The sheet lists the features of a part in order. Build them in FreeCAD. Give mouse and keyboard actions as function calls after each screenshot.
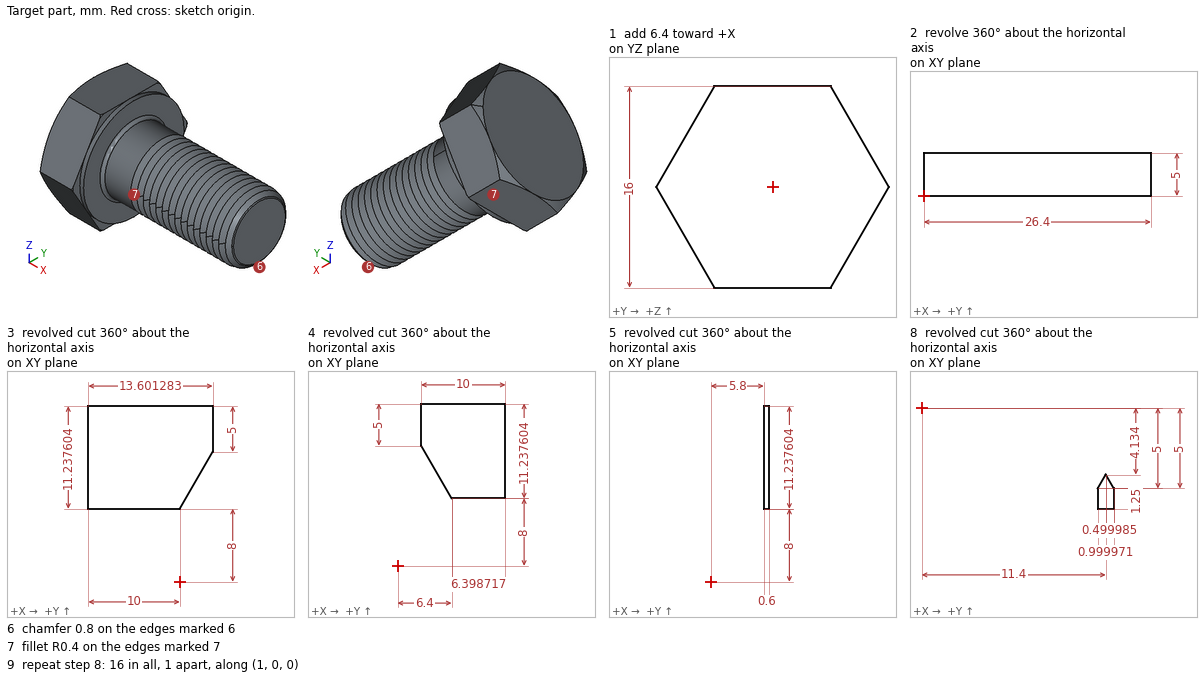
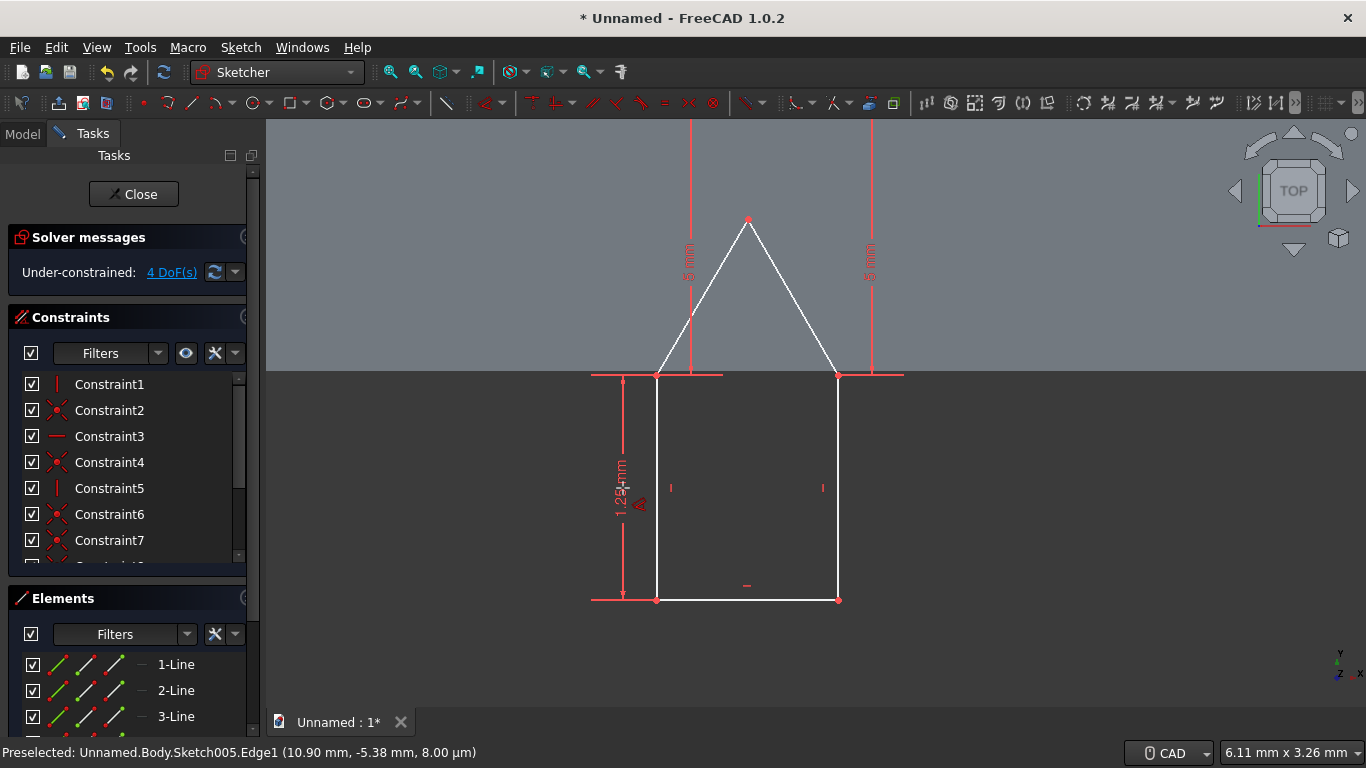
click(748, 220)
click(521, 254)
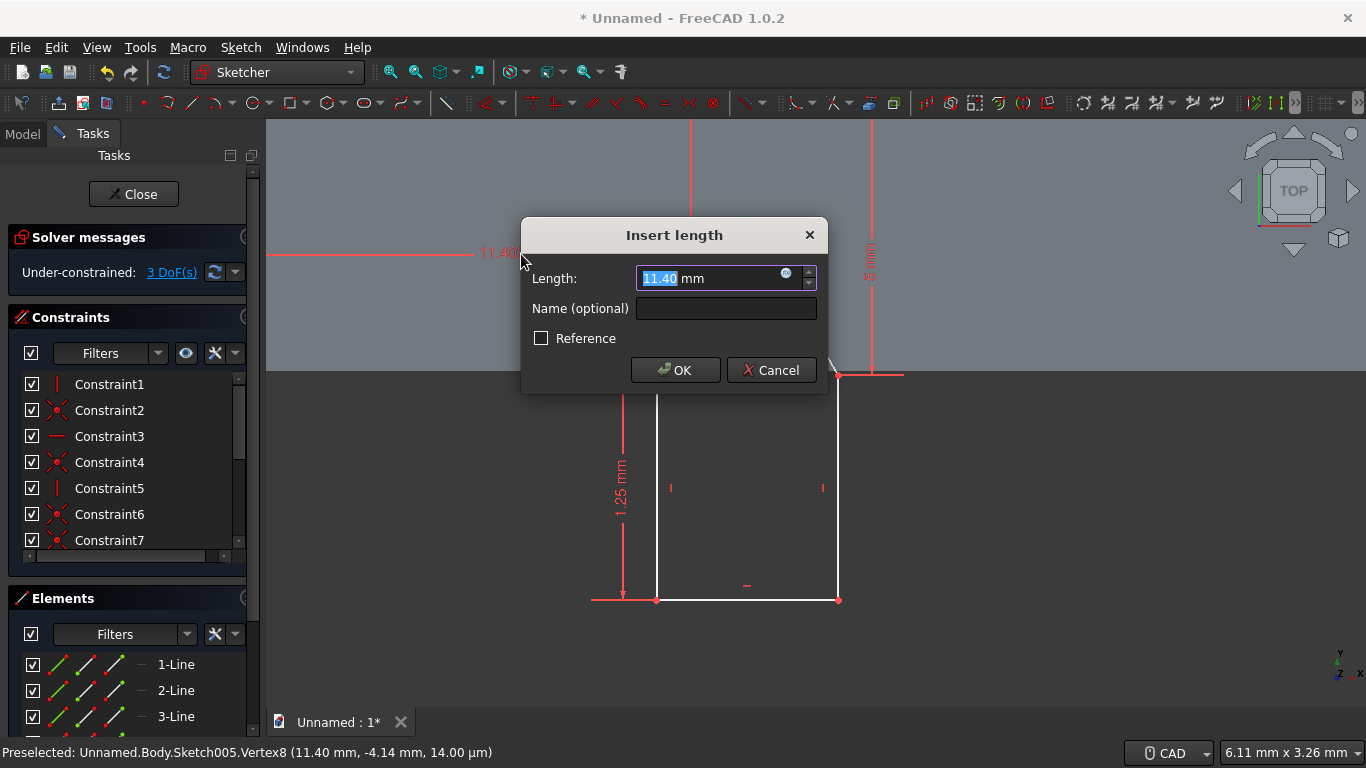
text(11.4)
key(Return)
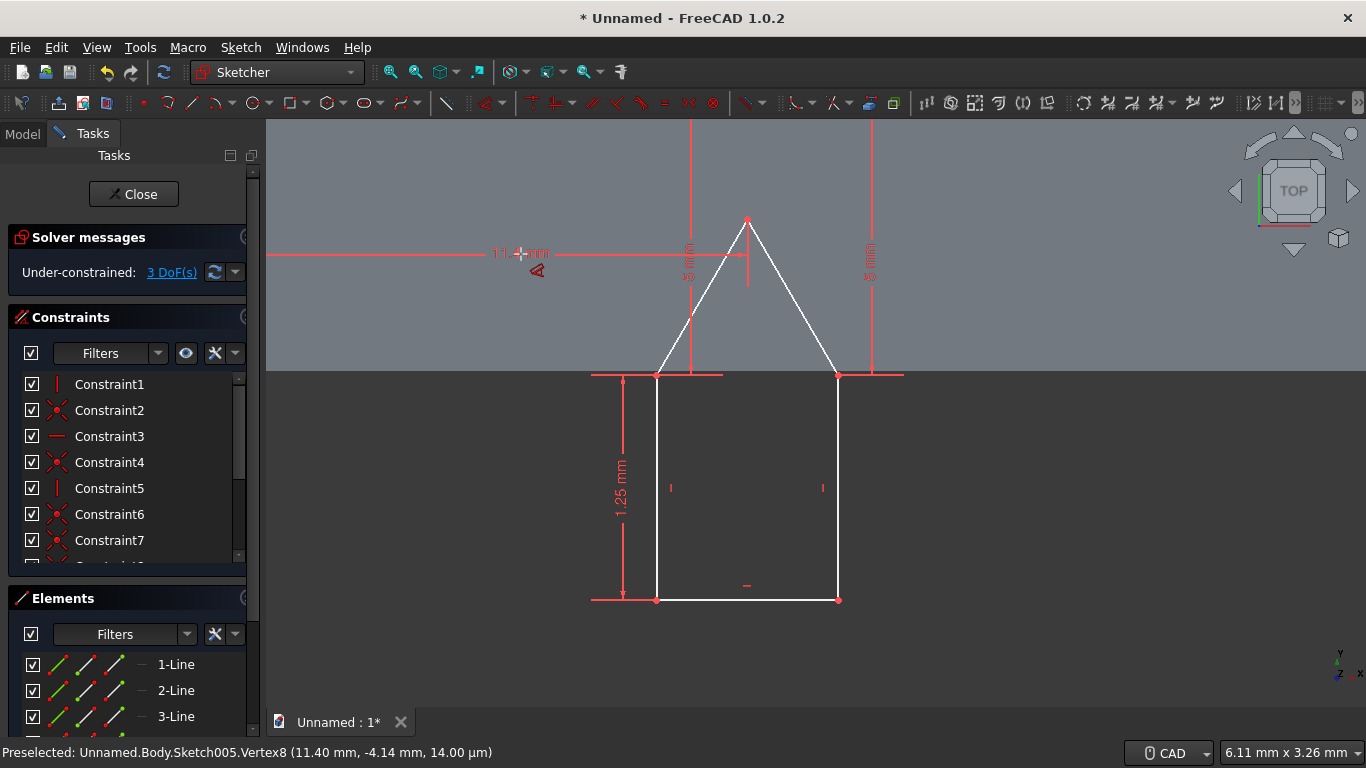
click(748, 220)
click(782, 183)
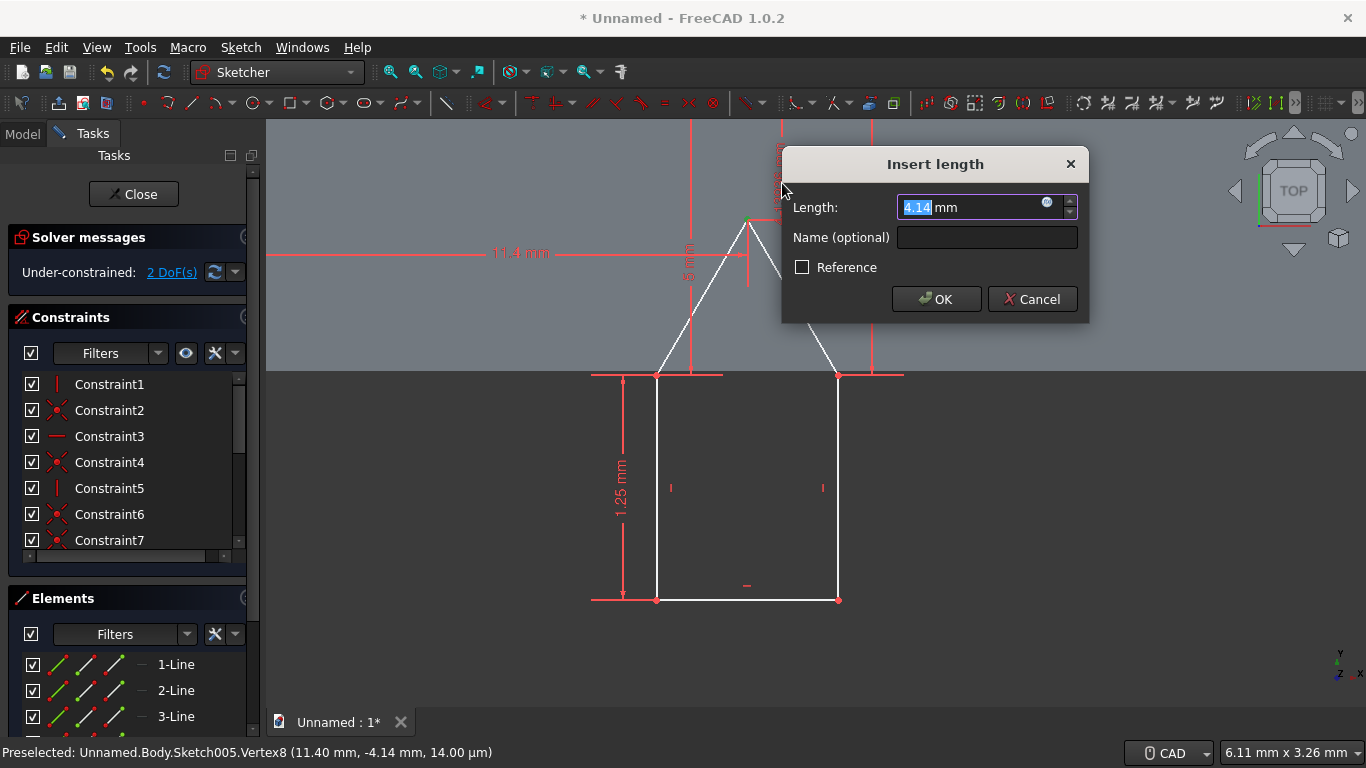
text(4.134)
key(Return)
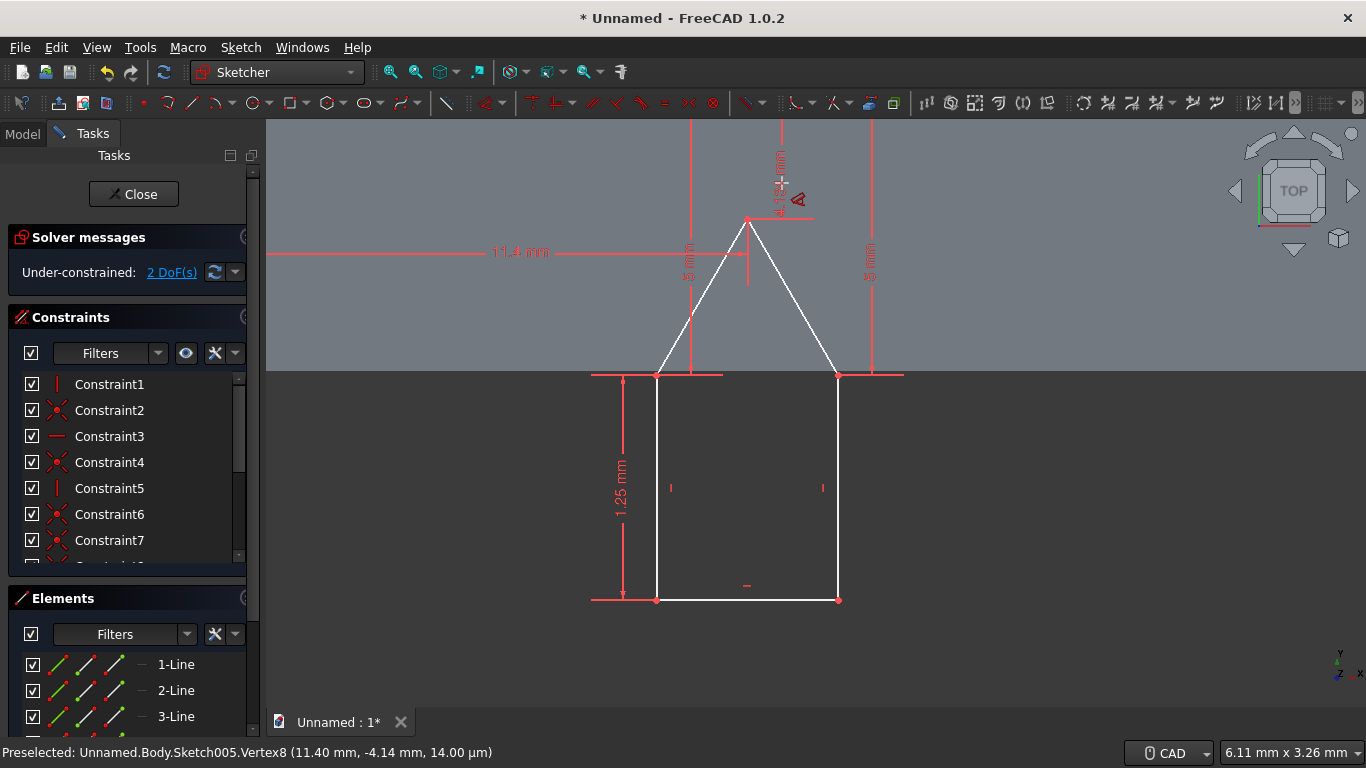
click(711, 600)
click(748, 634)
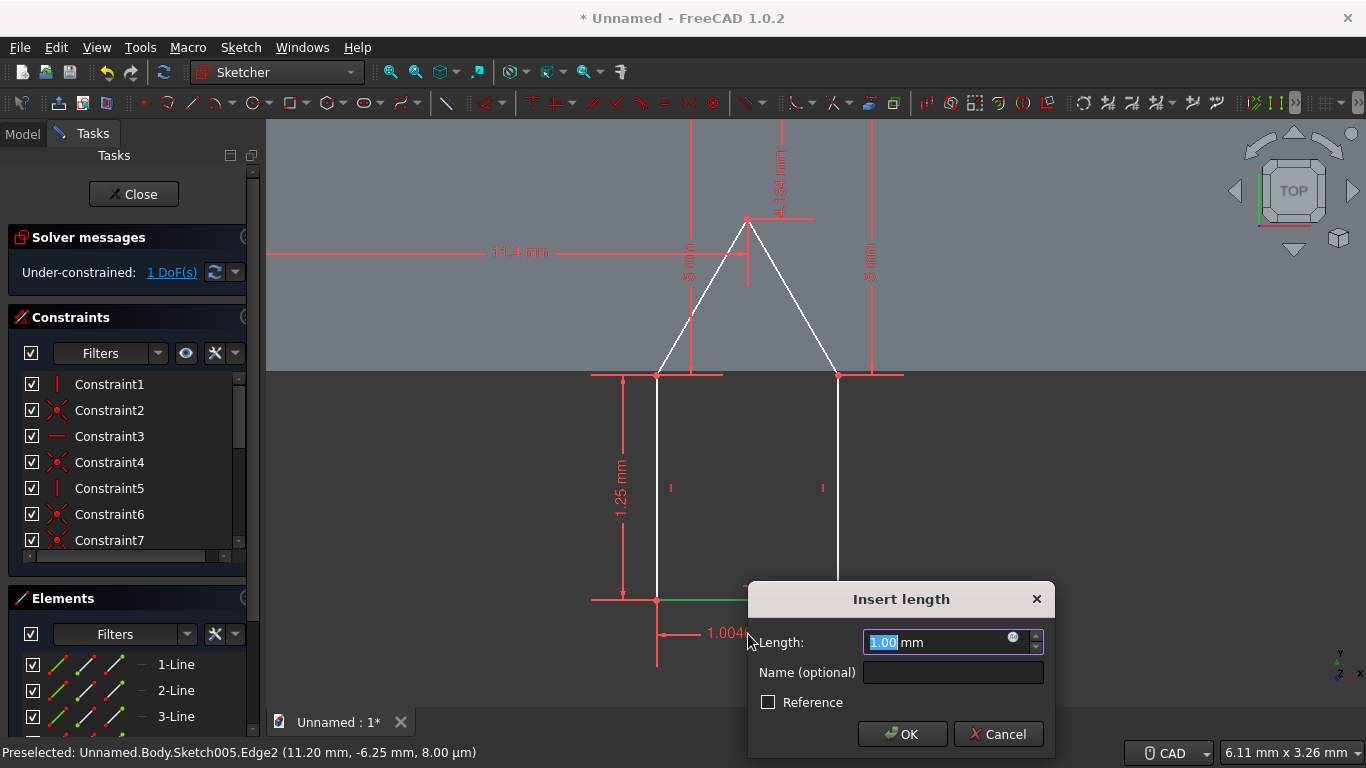
text(0.999971)
key(Return)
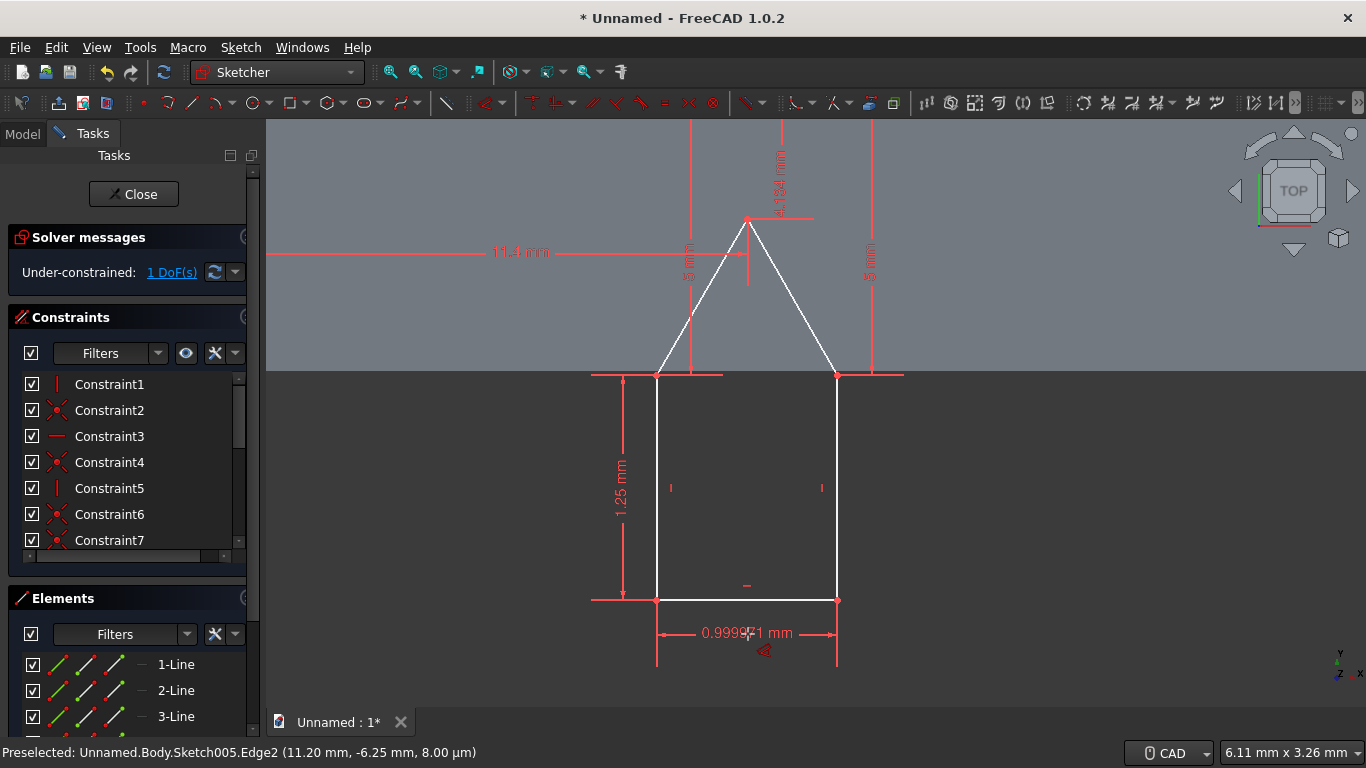
click(810, 328)
click(792, 409)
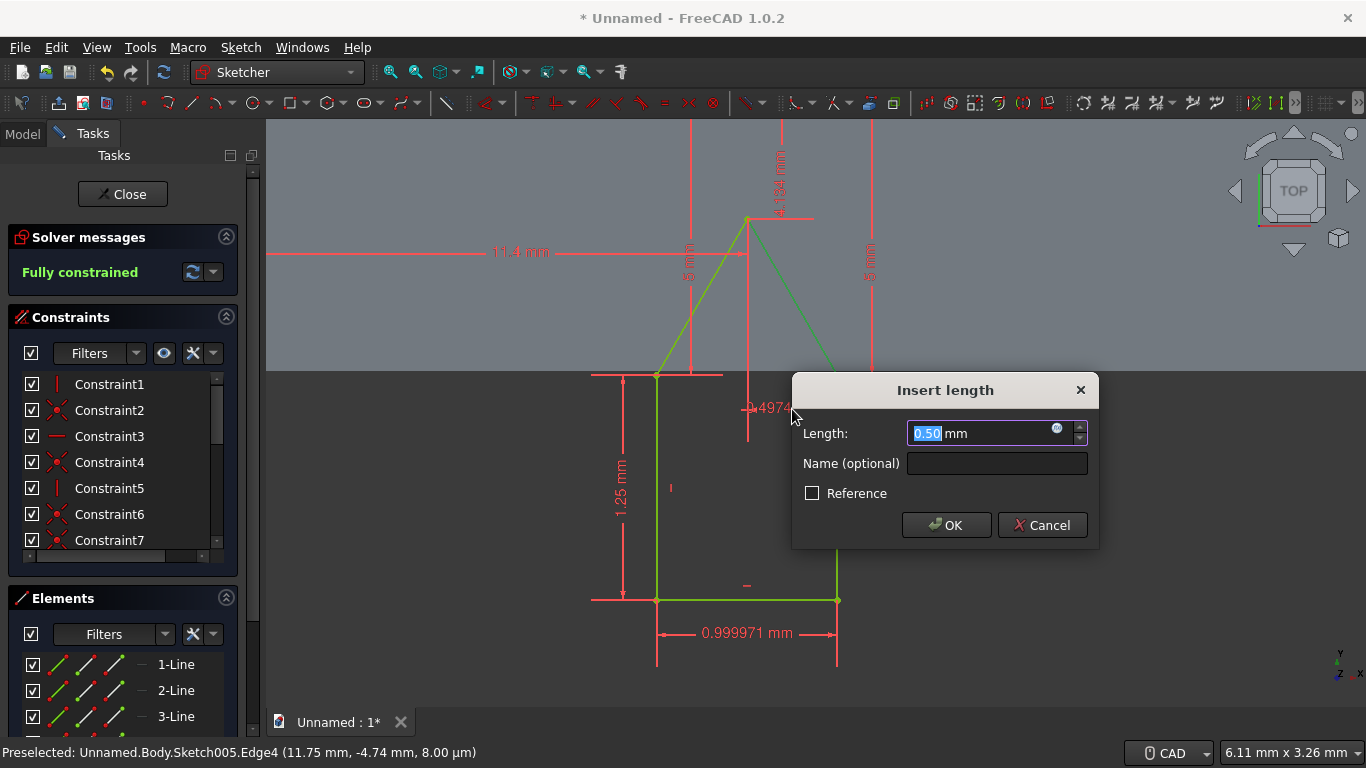
text(0.499985)
key(Return)
key(Escape)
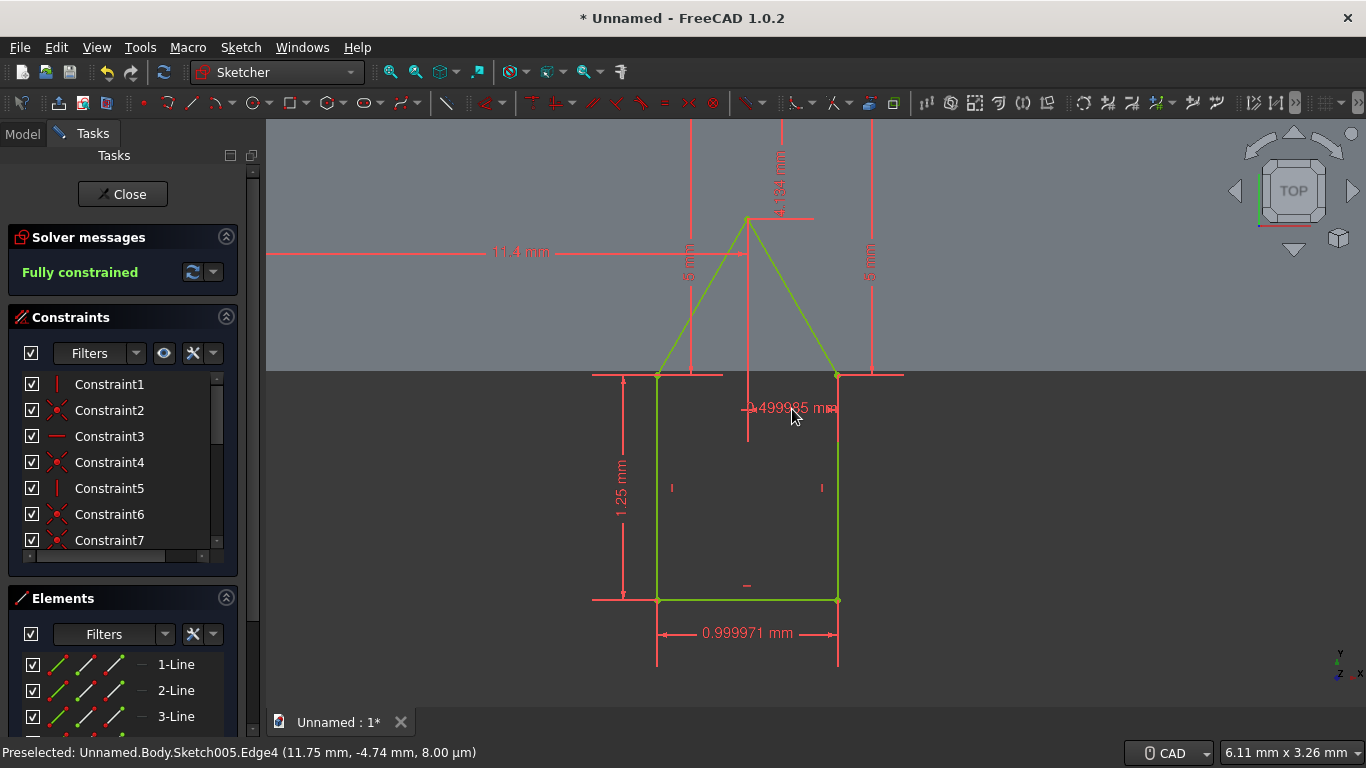
click(123, 194)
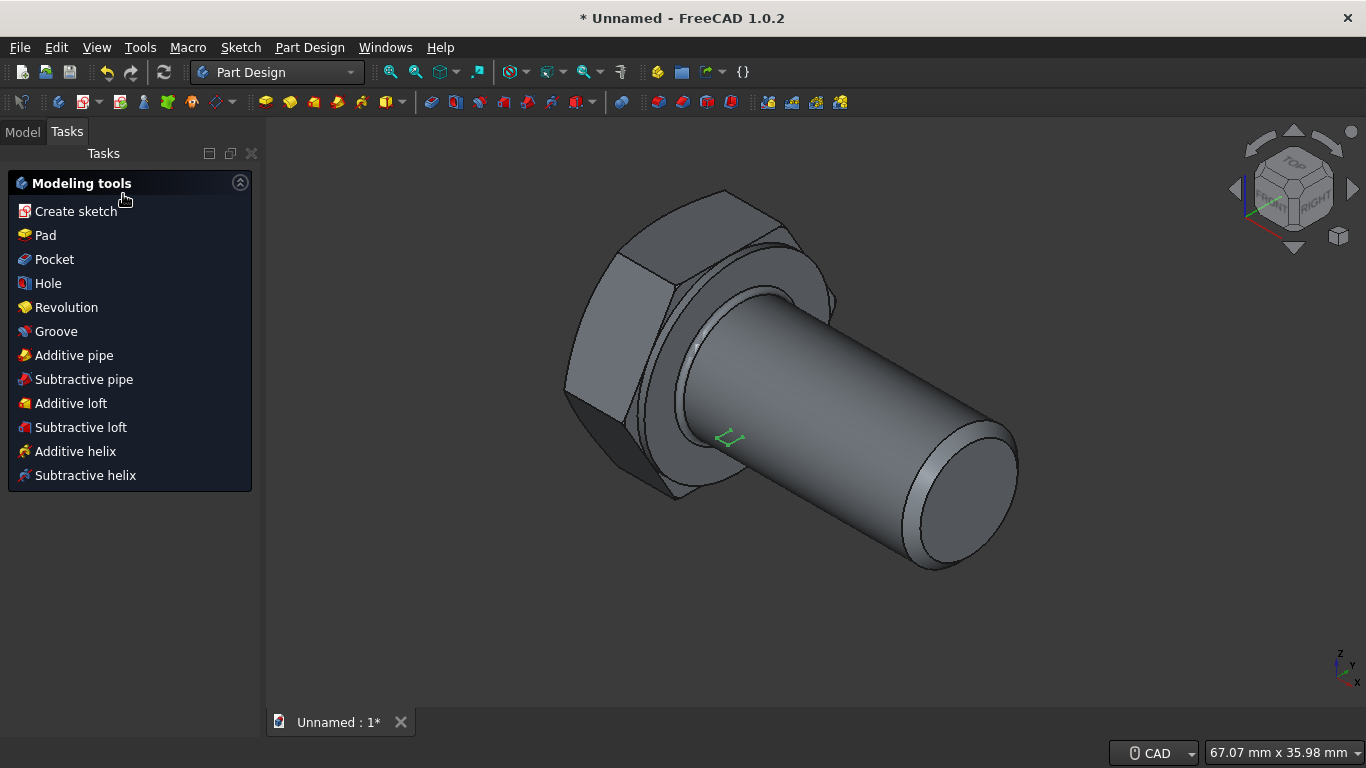
click(480, 102)